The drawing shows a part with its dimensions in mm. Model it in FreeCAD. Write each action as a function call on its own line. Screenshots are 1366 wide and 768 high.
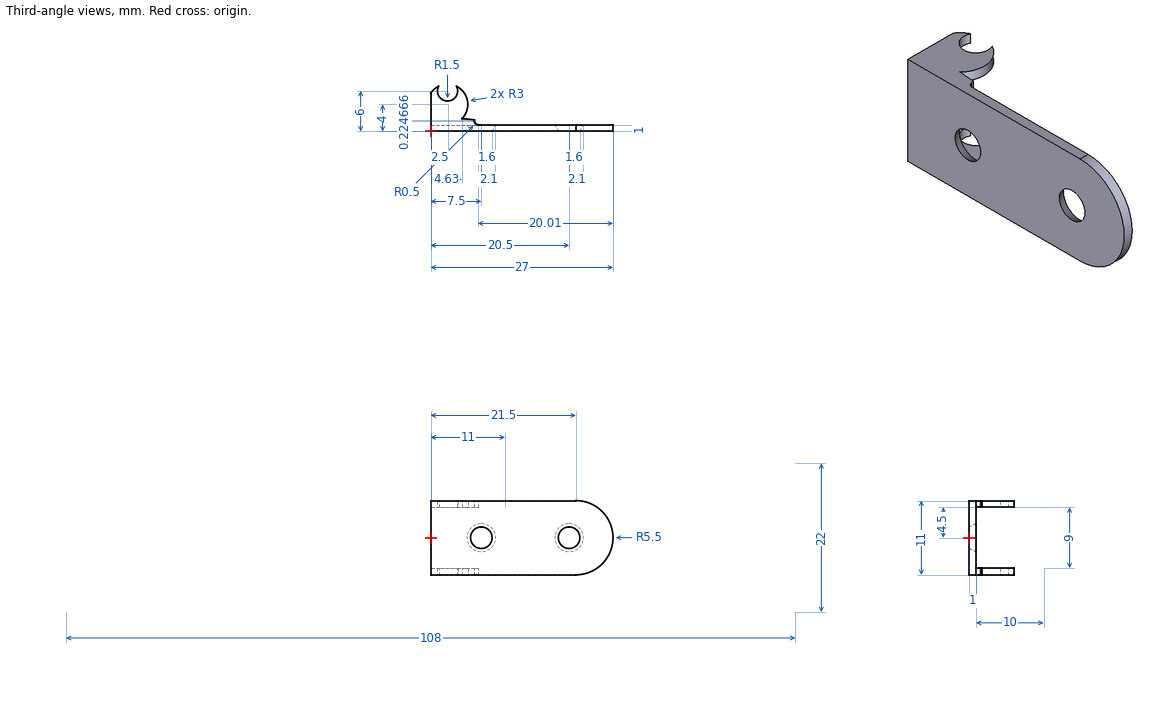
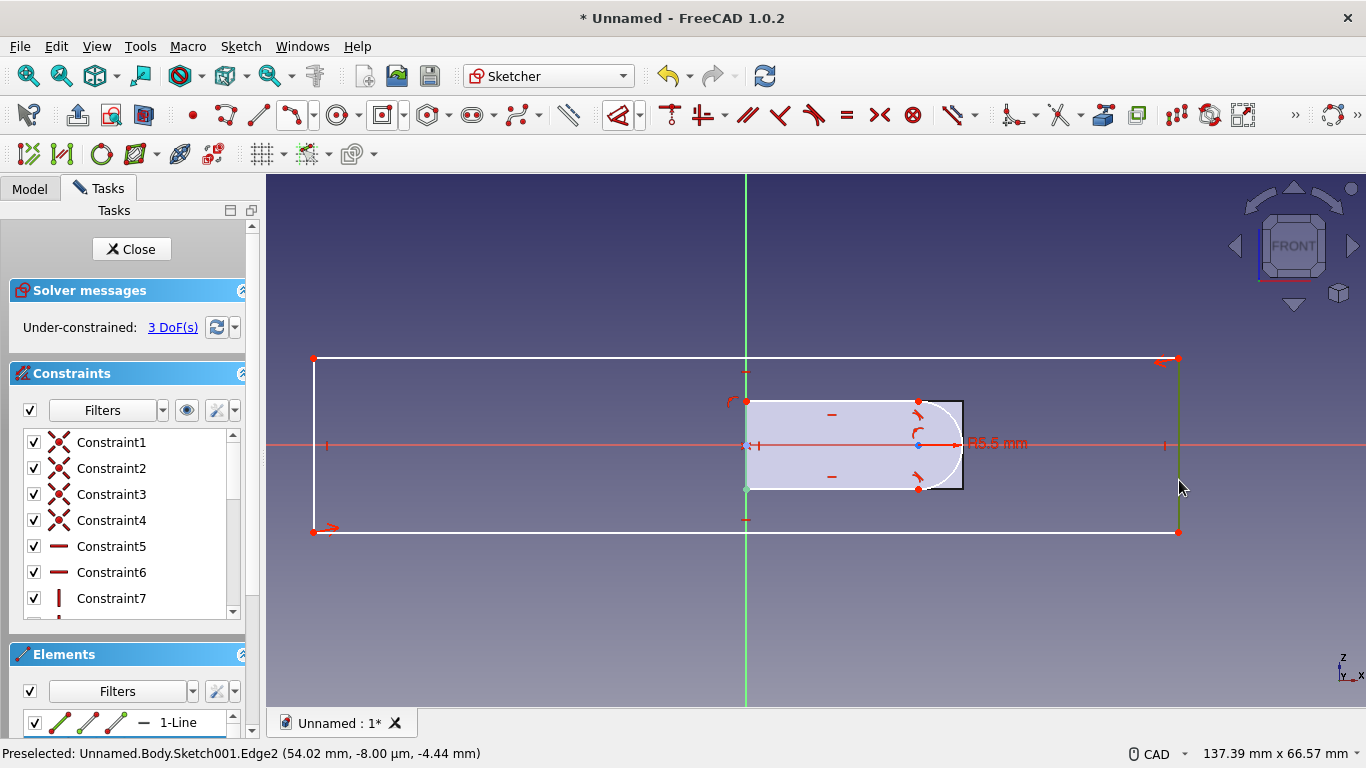
key(i)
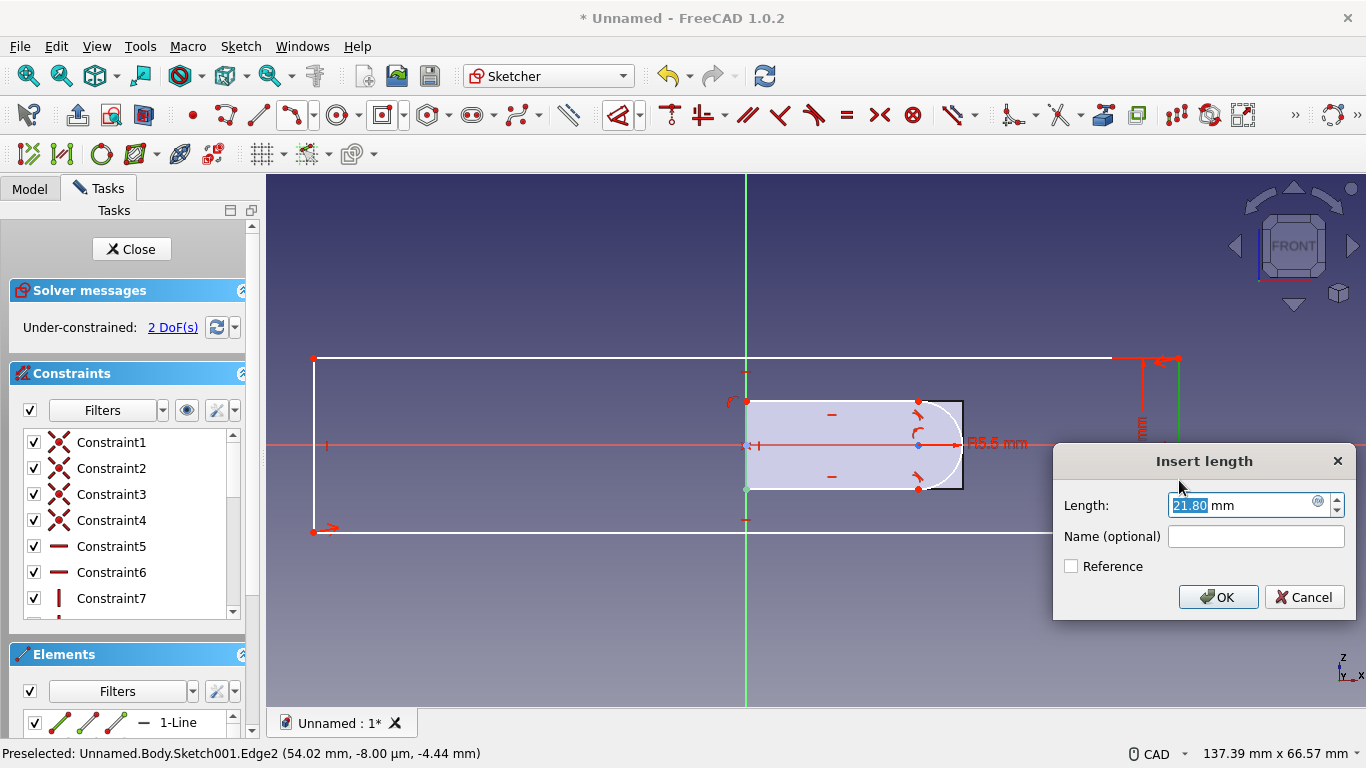
text(22)
key(Return)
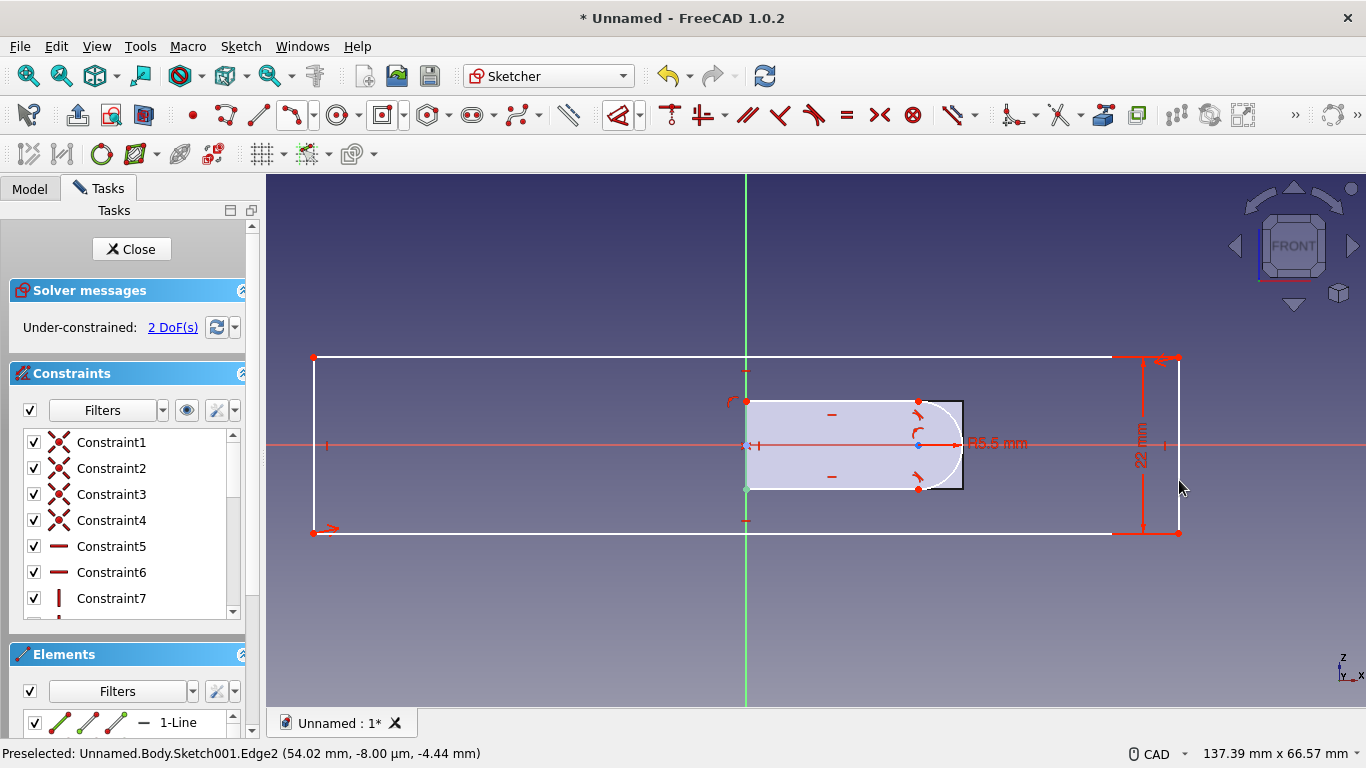
click(573, 533)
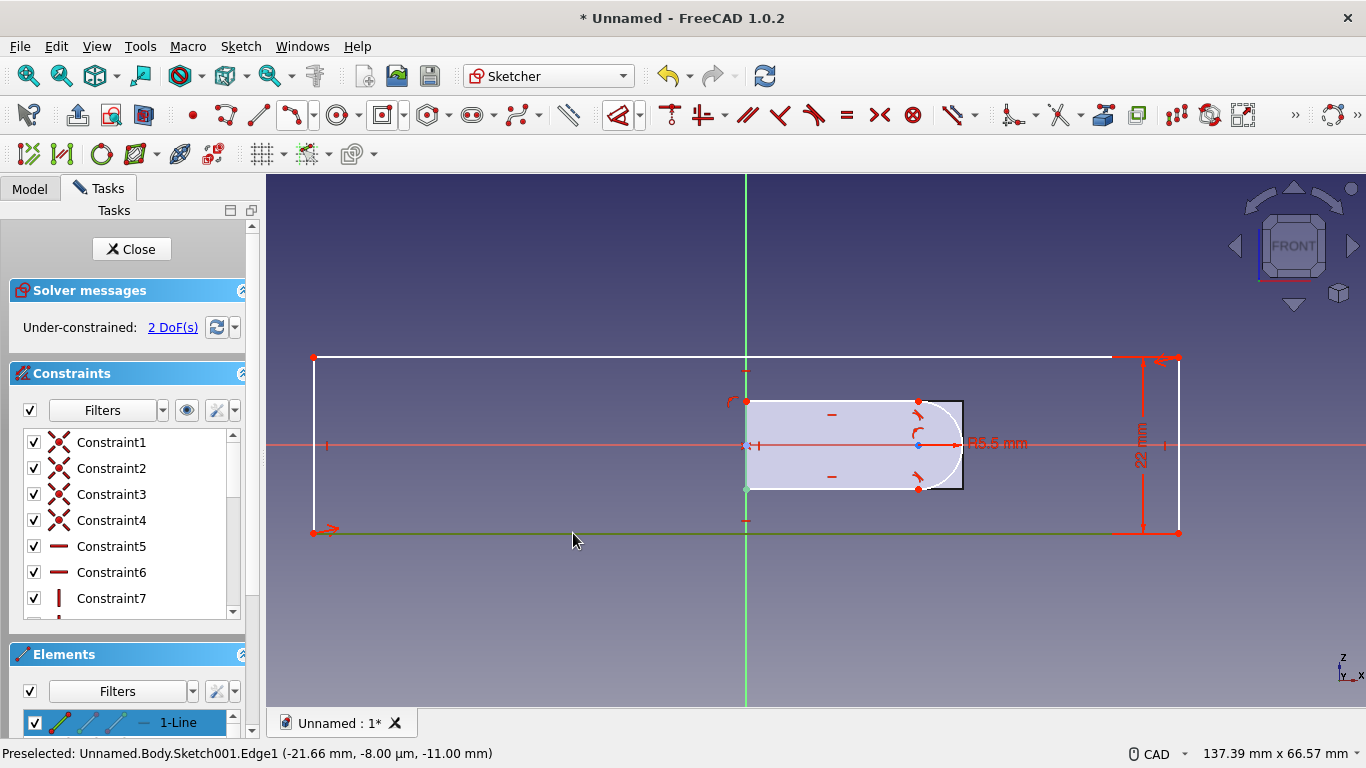
key(l)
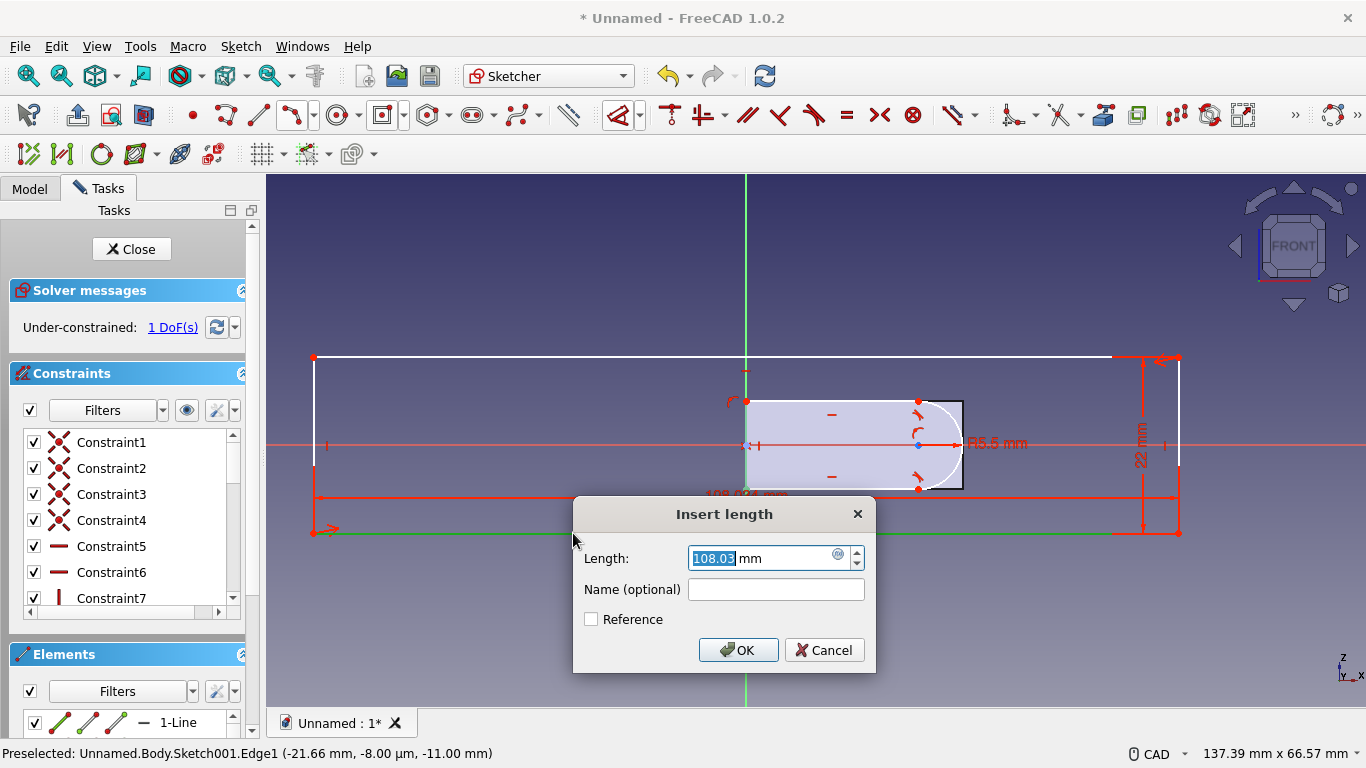
text(108)
key(Return)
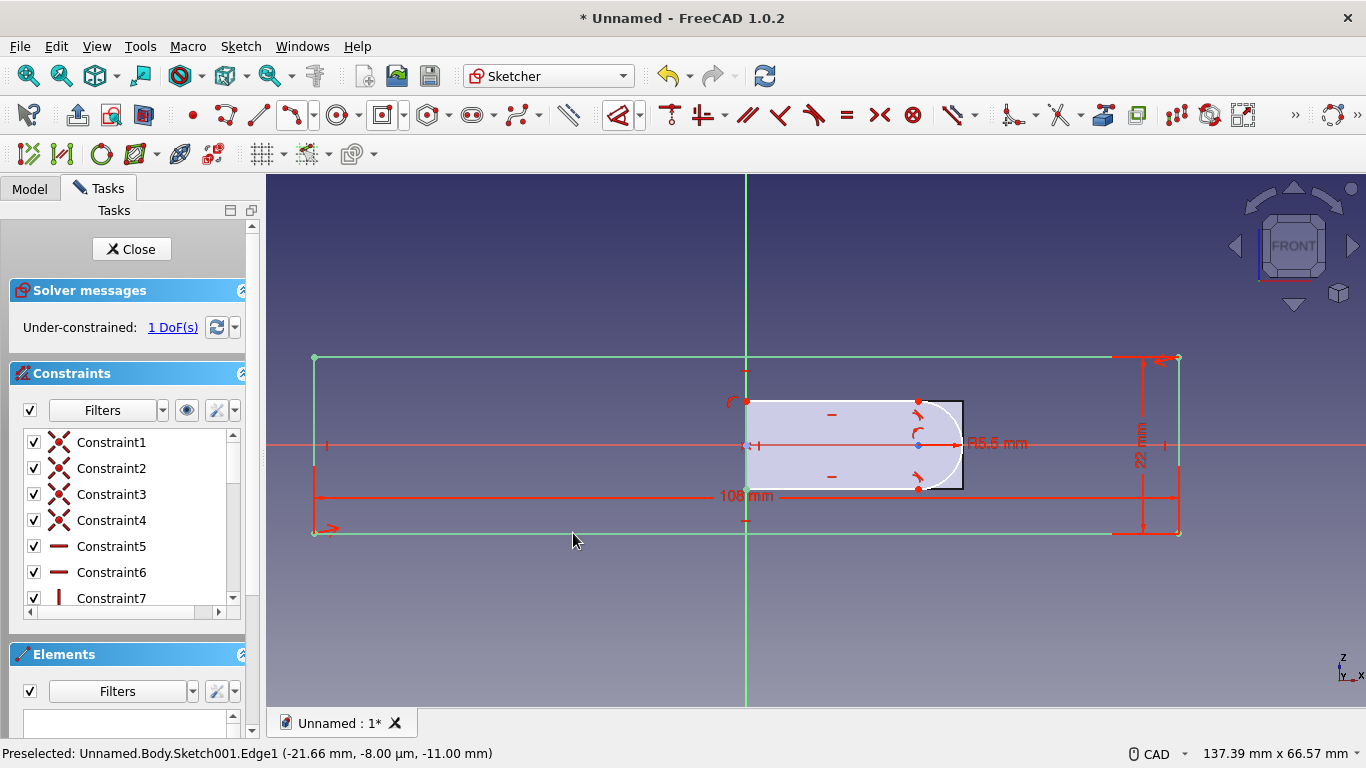
click(867, 401)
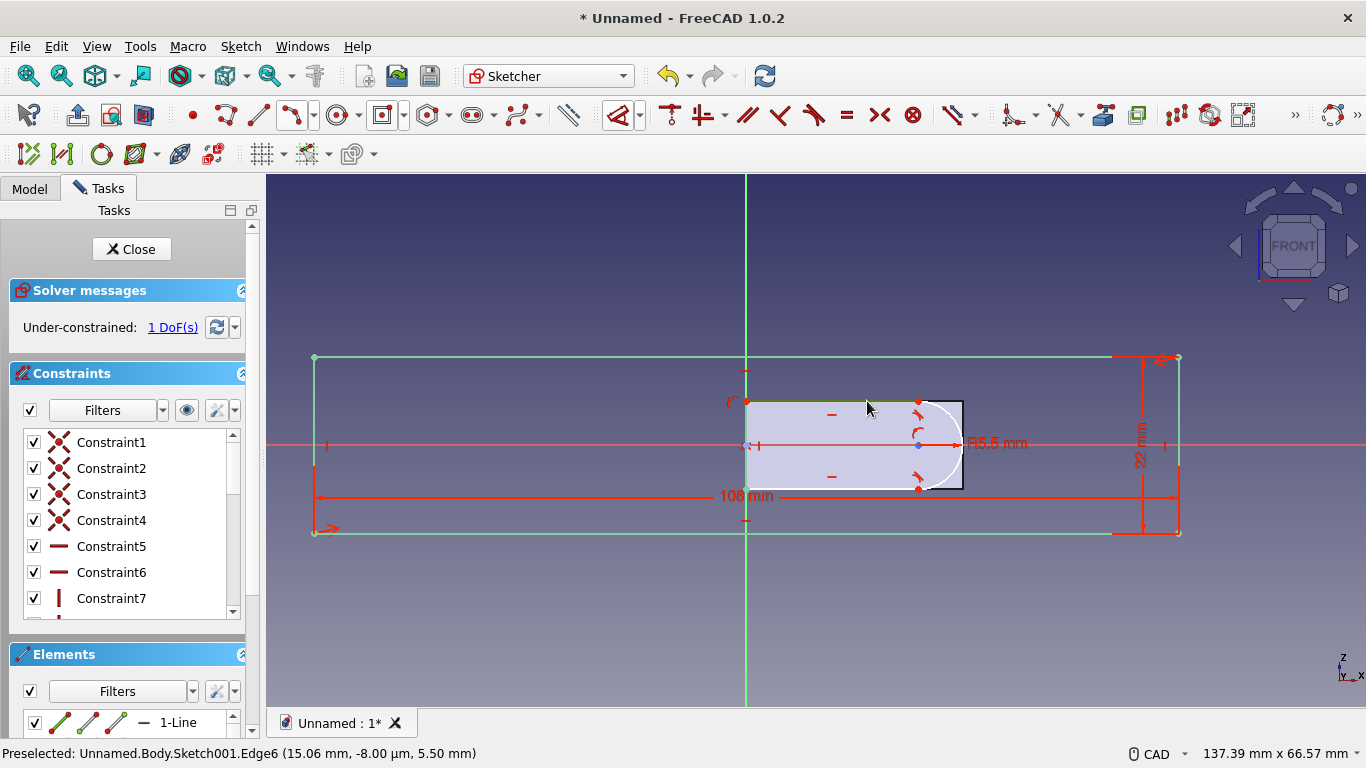
key(l)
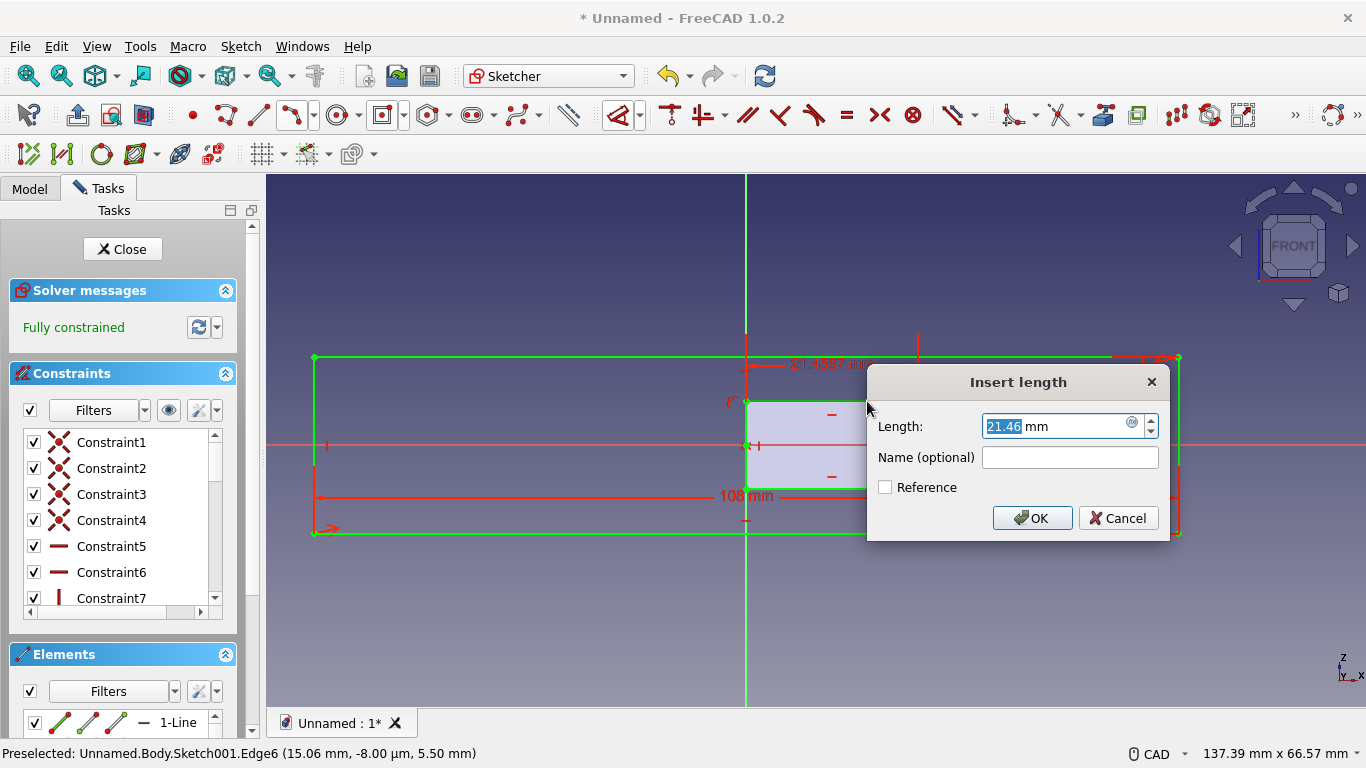
text(21.5)
key(Return)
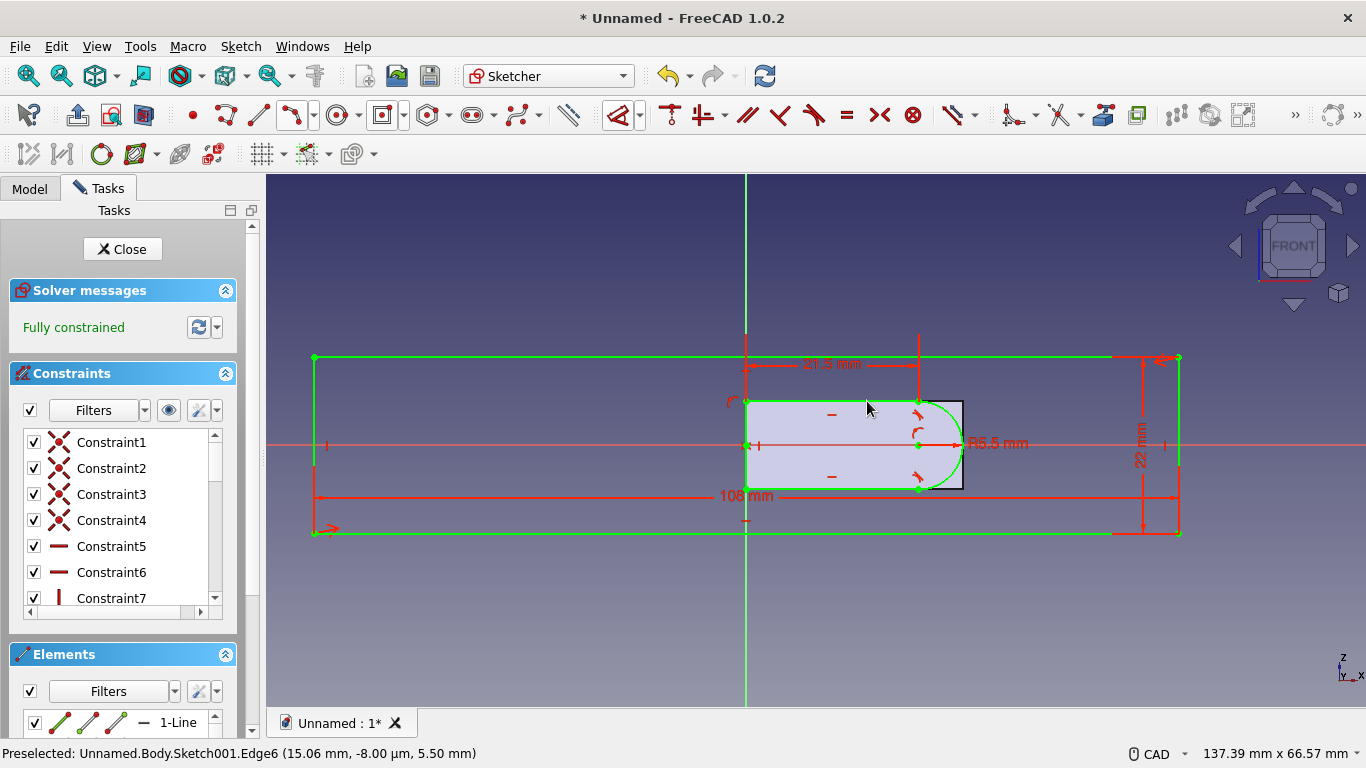
click(123, 249)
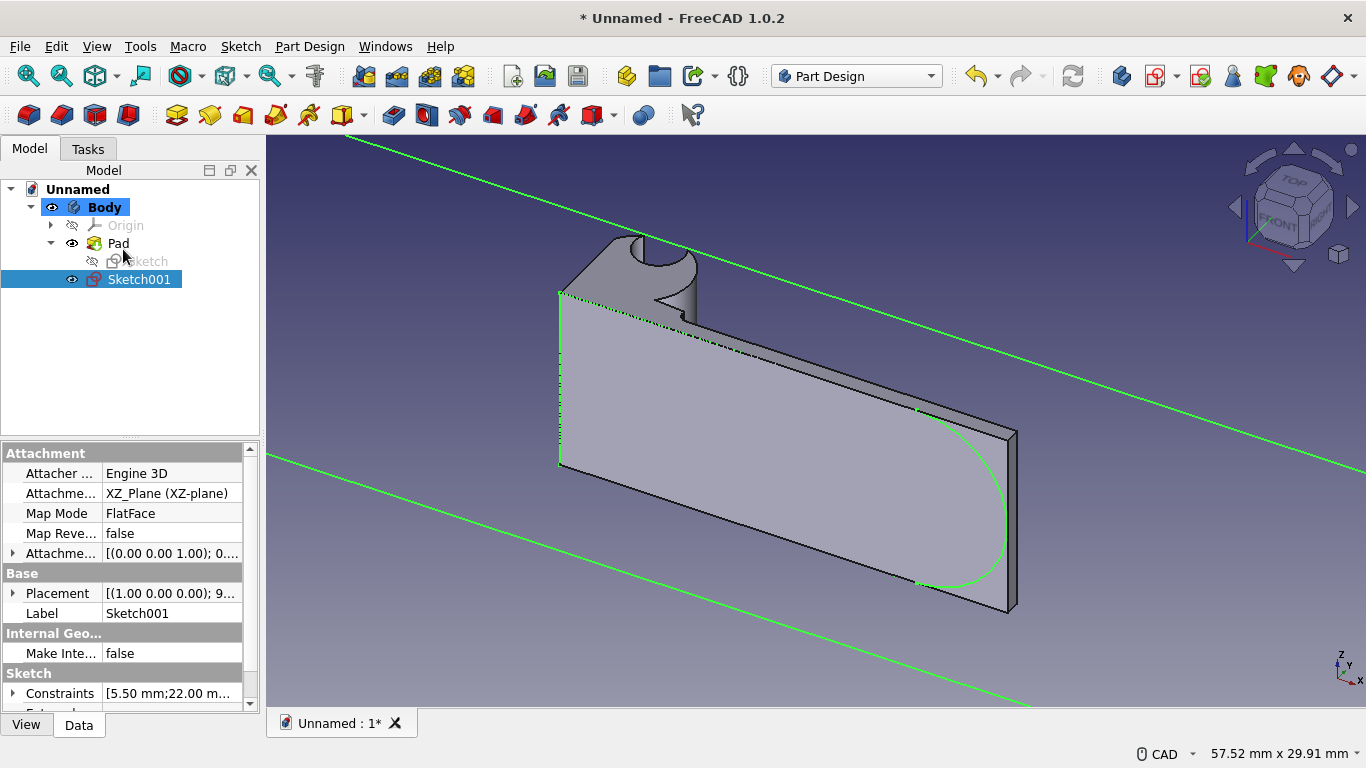
click(394, 116)